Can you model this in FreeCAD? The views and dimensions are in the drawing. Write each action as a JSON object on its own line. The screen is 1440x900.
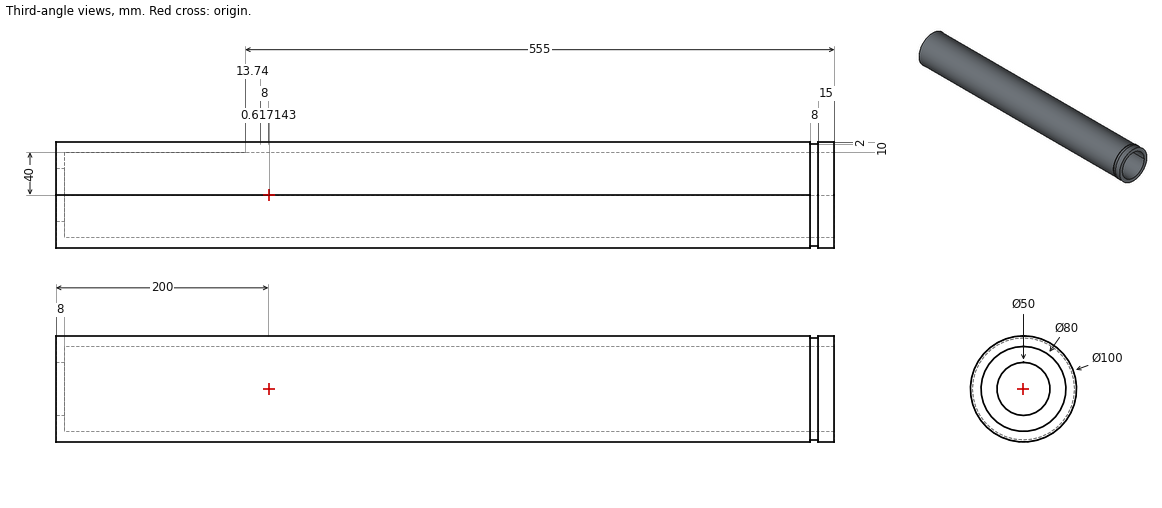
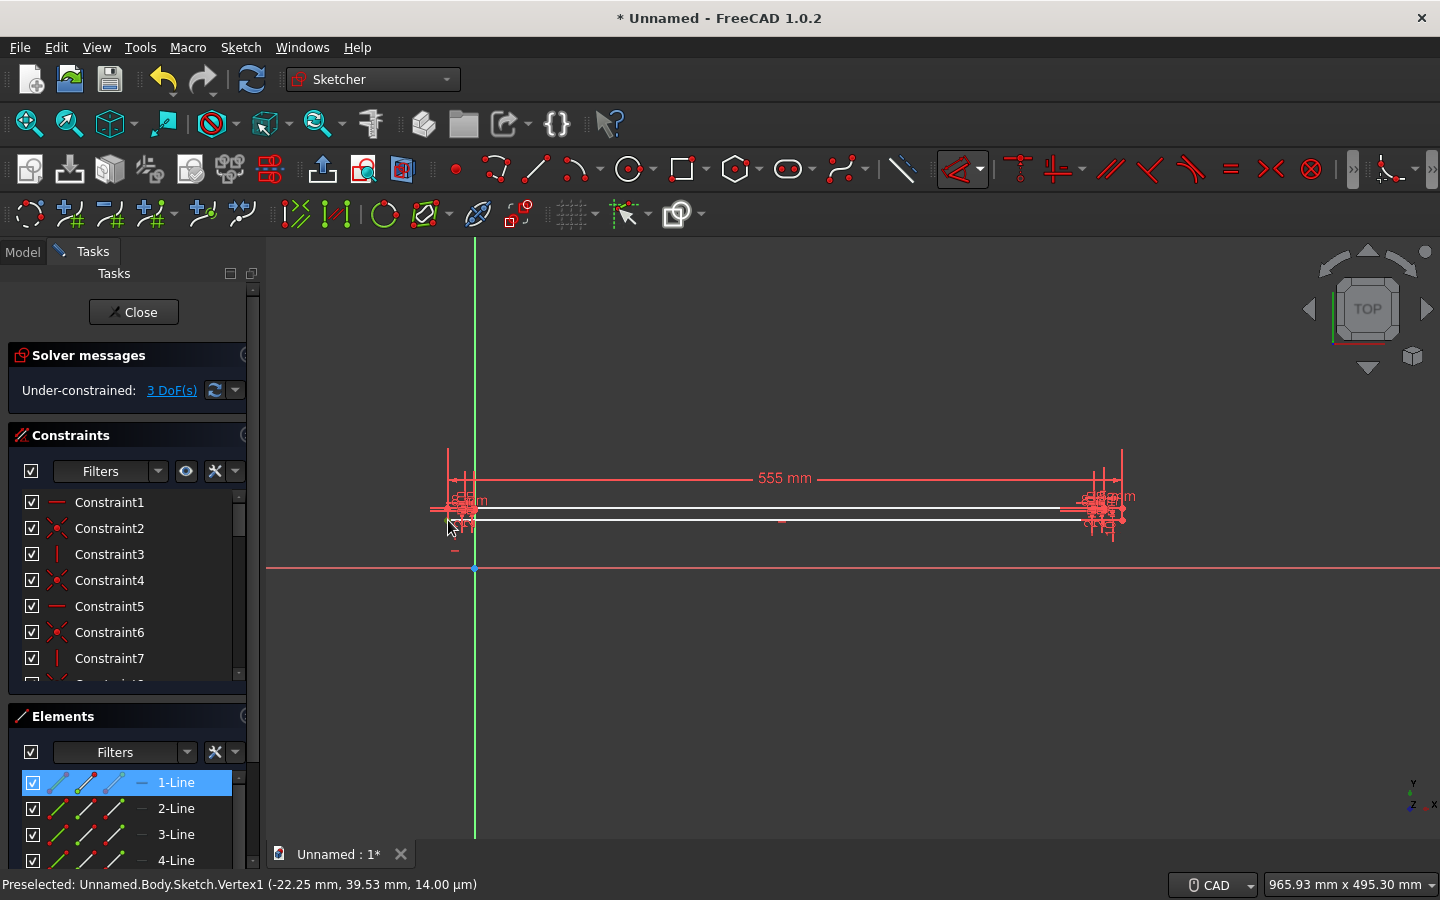
{"action": "key", "text": "i"}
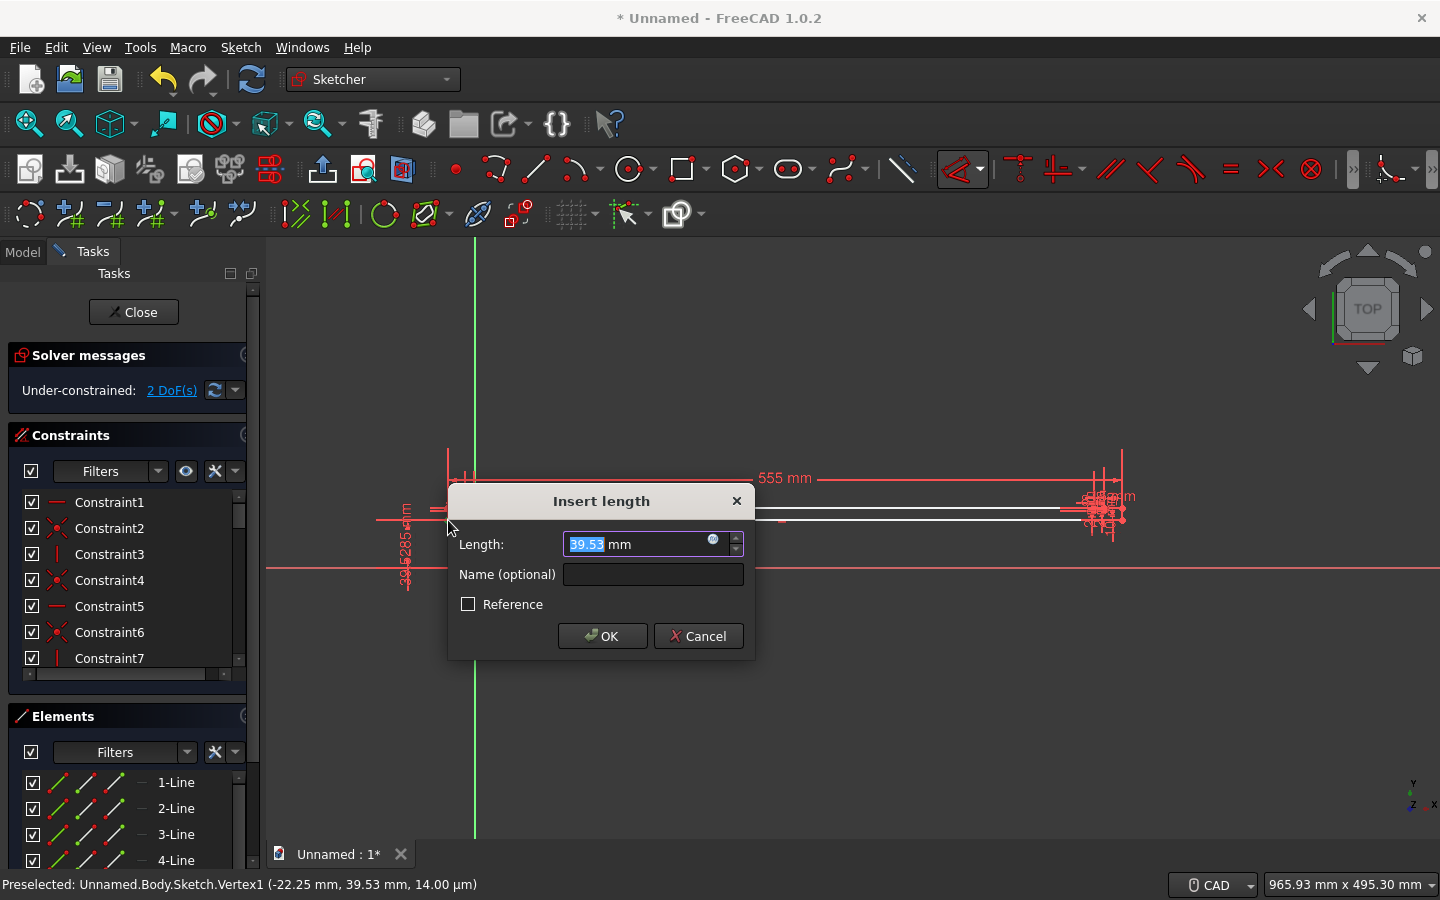
{"action": "type", "text": "40"}
{"action": "key", "text": "Return"}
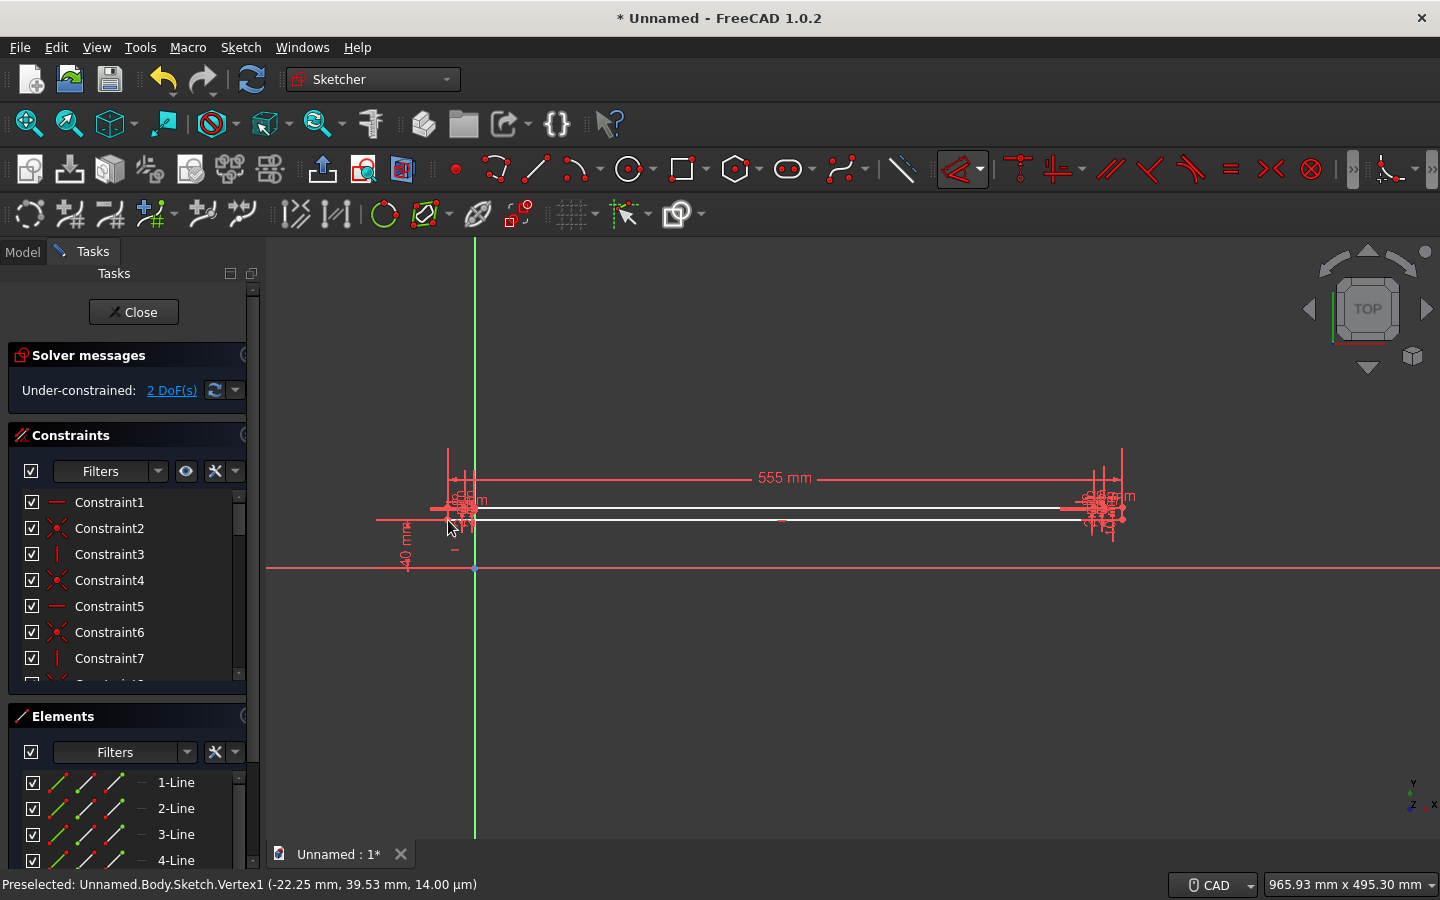
{"action": "scroll", "coordinate": [456, 508], "scroll_direction": "up", "scroll_amount": 5}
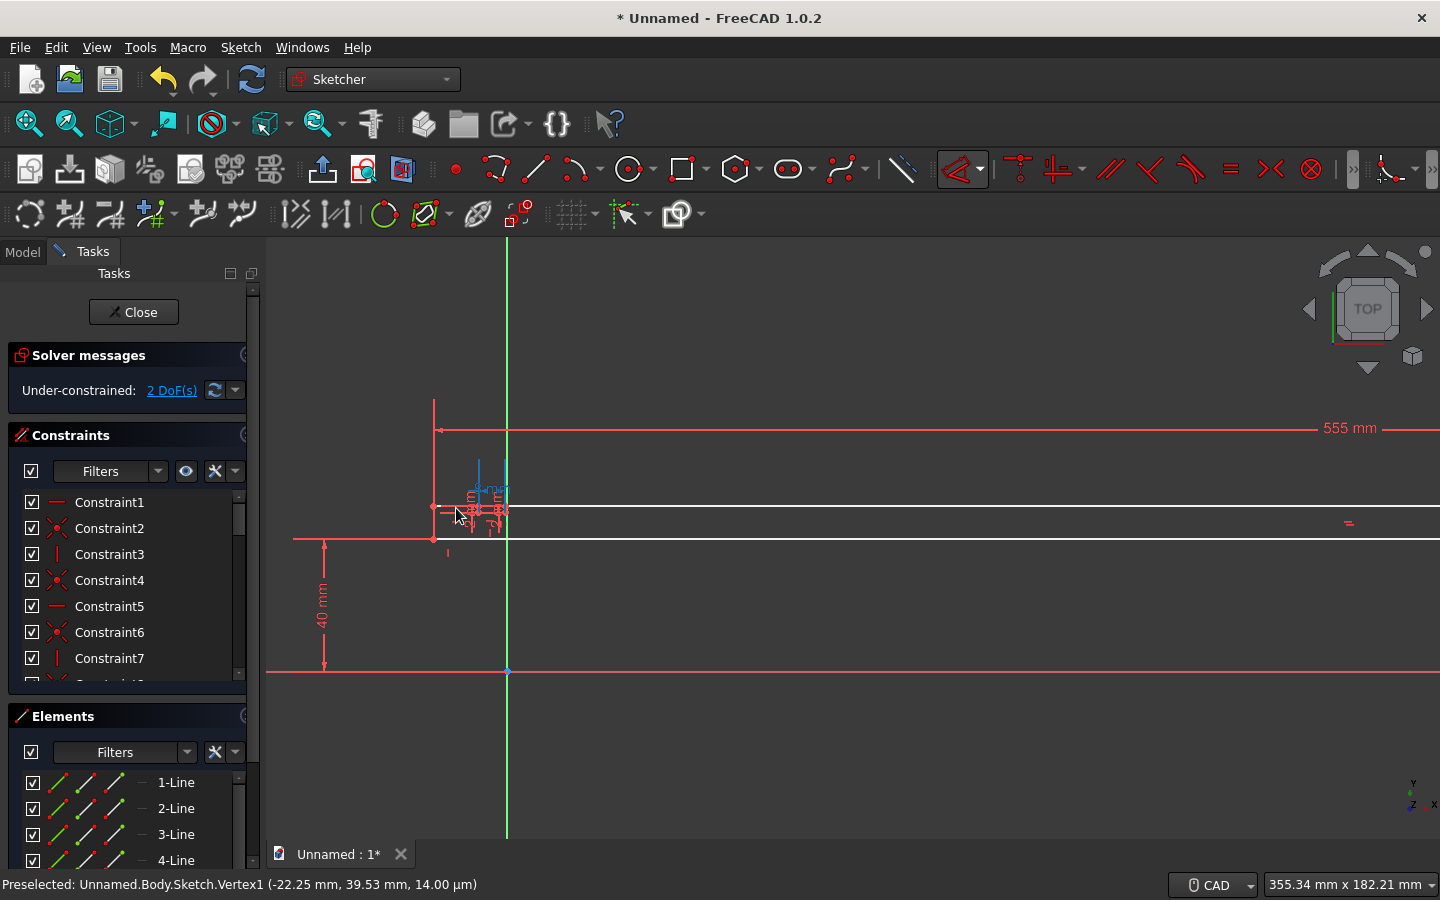
{"action": "left_click", "coordinate": [456, 506]}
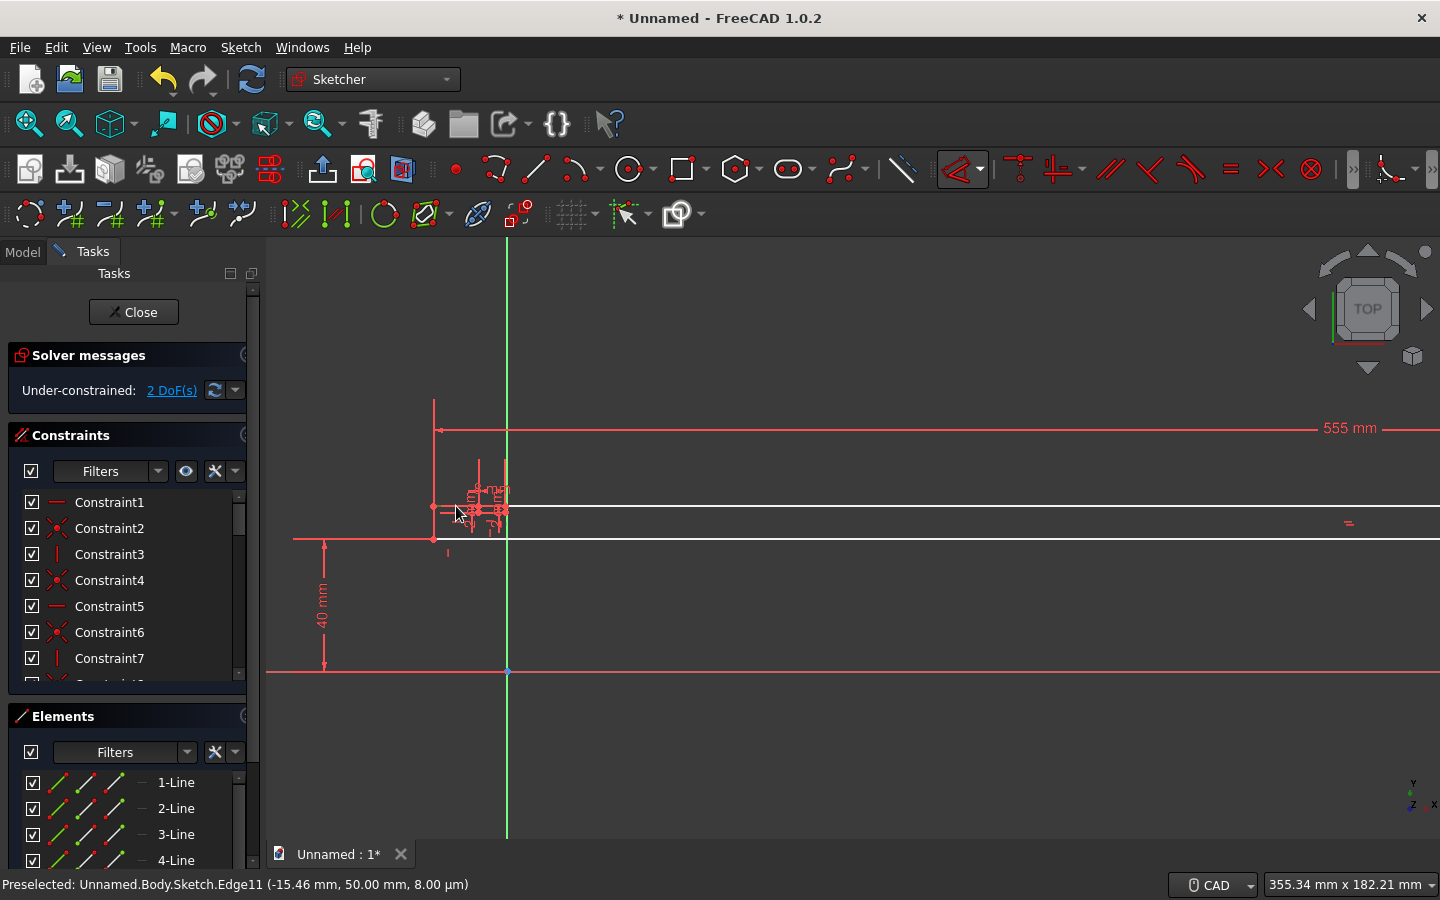
{"action": "key", "text": "l"}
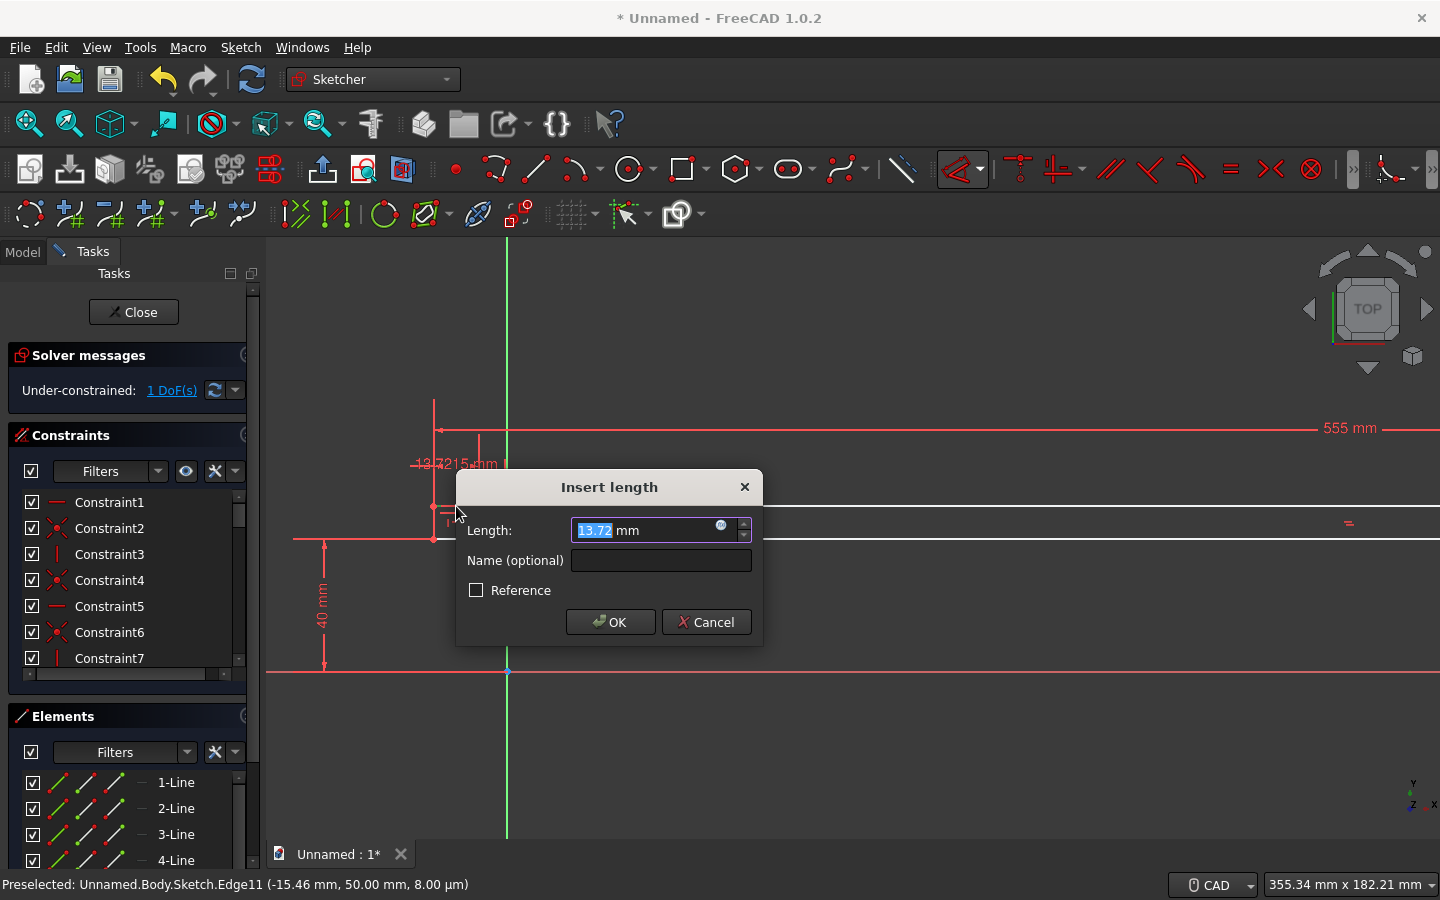
{"action": "type", "text": "13.74"}
{"action": "key", "text": "Return"}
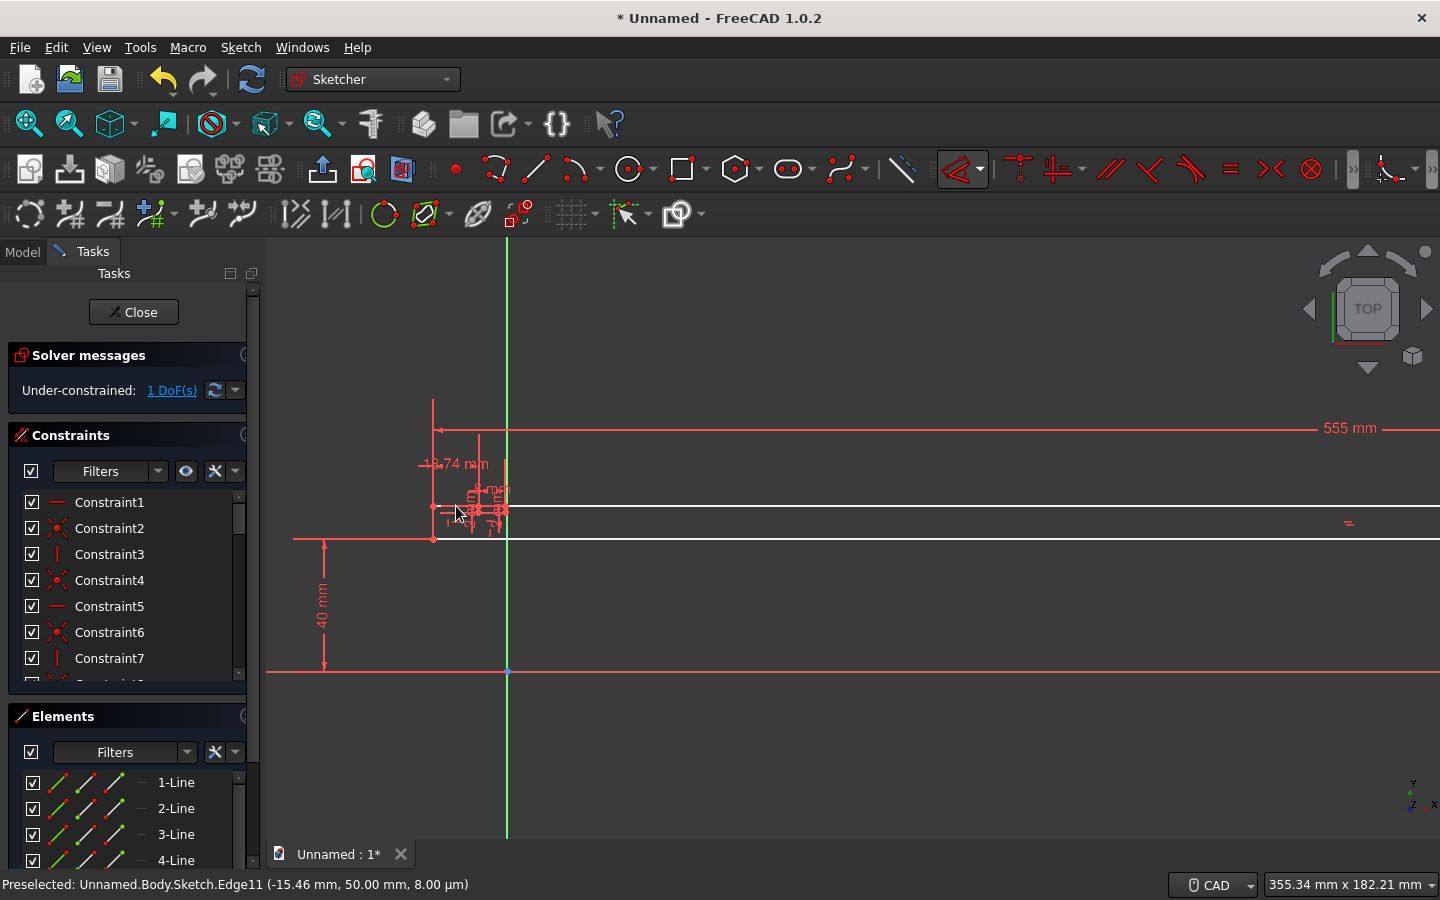
{"action": "scroll", "coordinate": [505, 506], "scroll_direction": "up", "scroll_amount": 15}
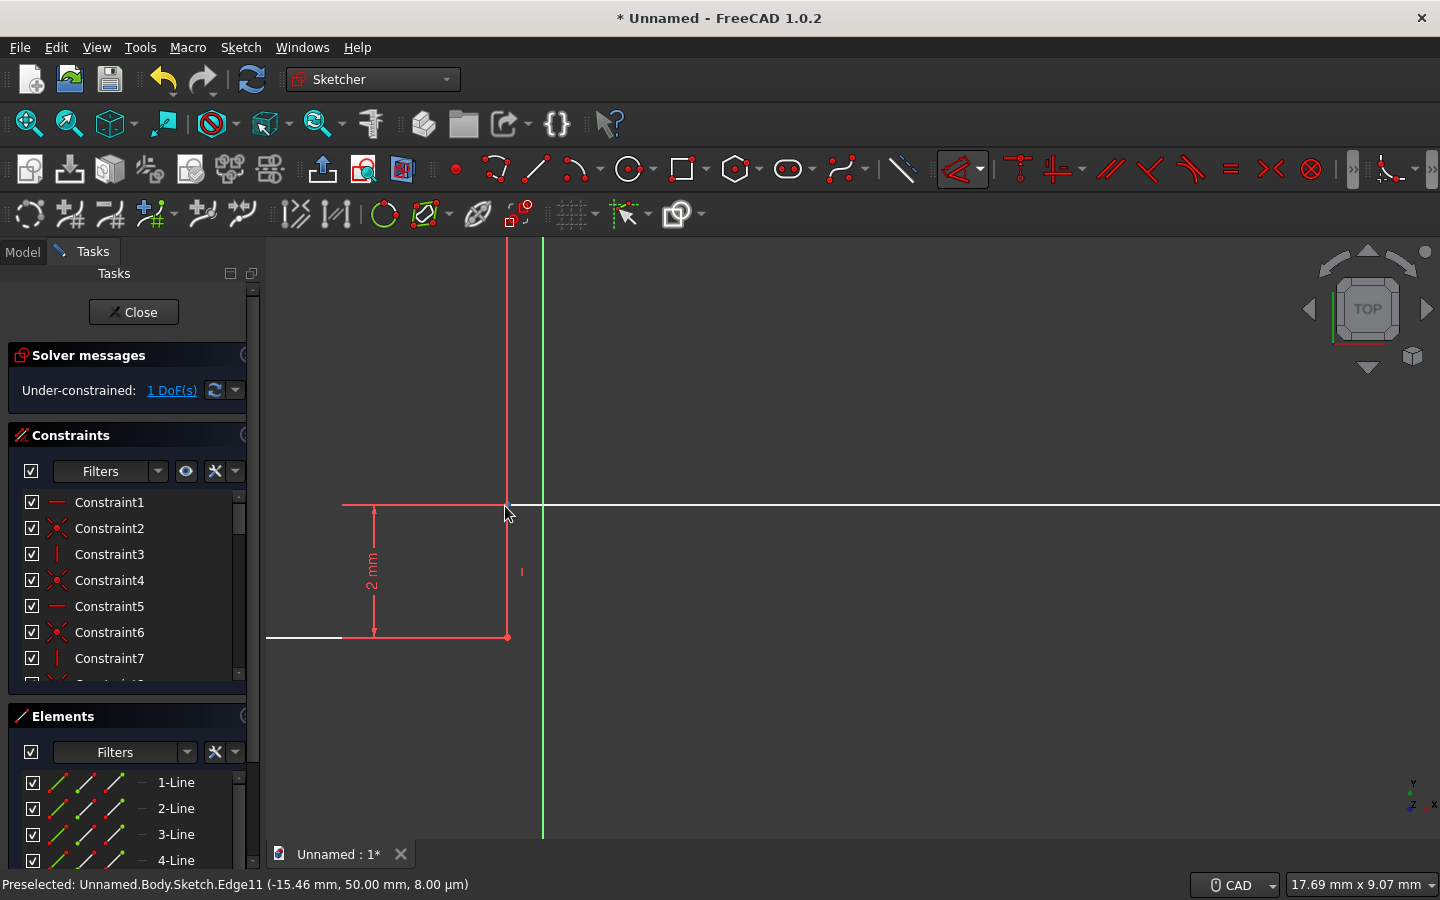
{"action": "left_click", "coordinate": [507, 505]}